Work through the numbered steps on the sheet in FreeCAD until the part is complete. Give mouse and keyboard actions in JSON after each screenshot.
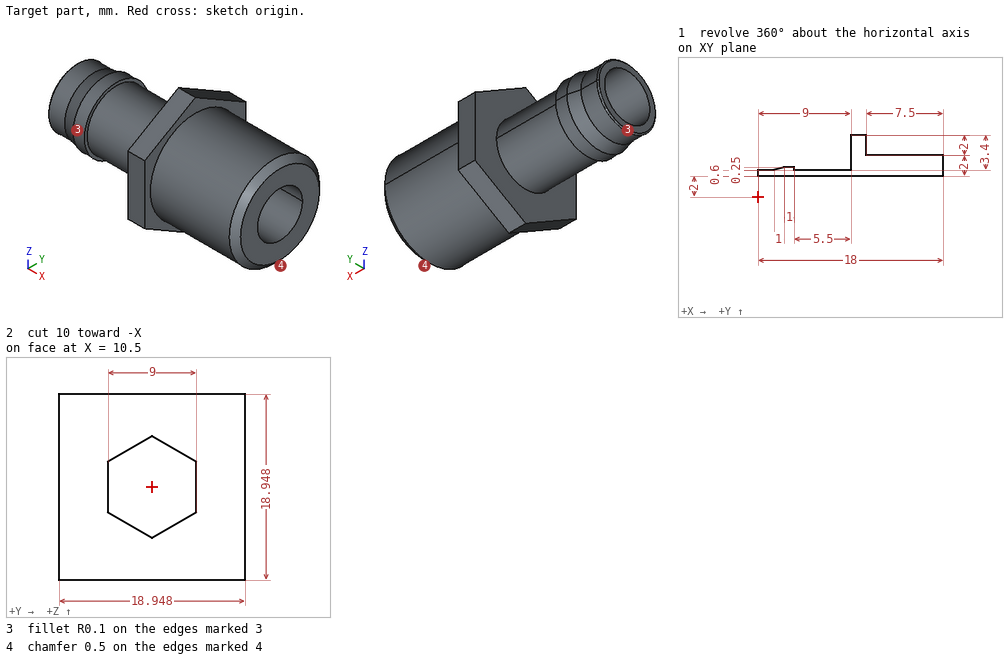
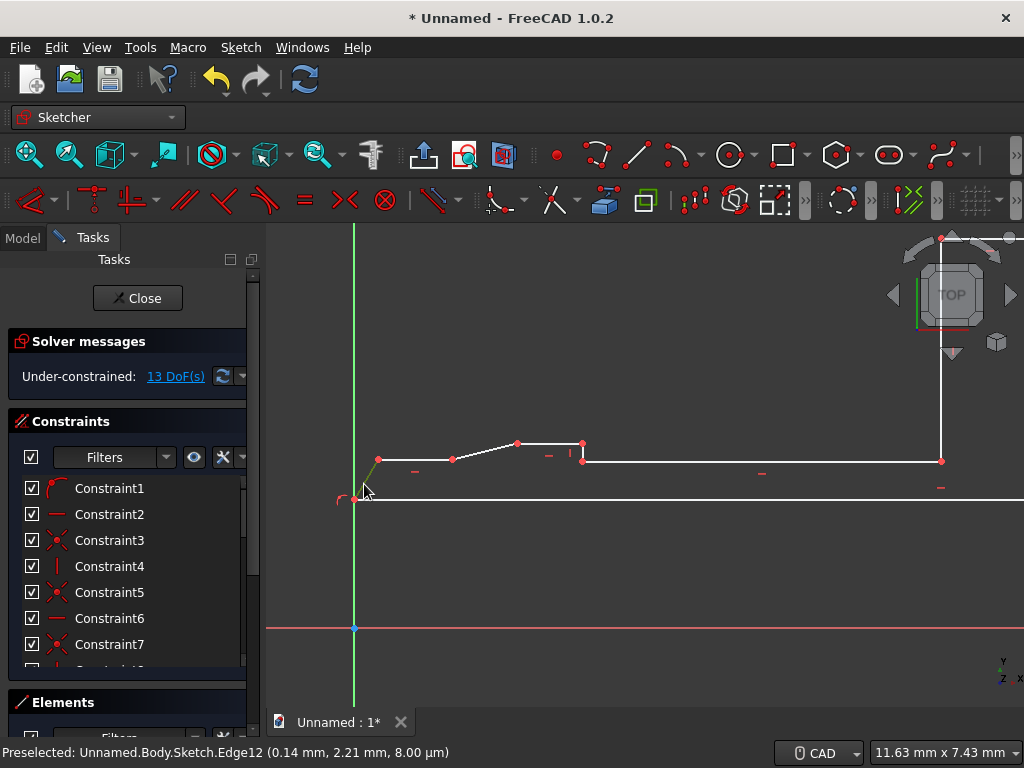
{"action": "key", "text": "v"}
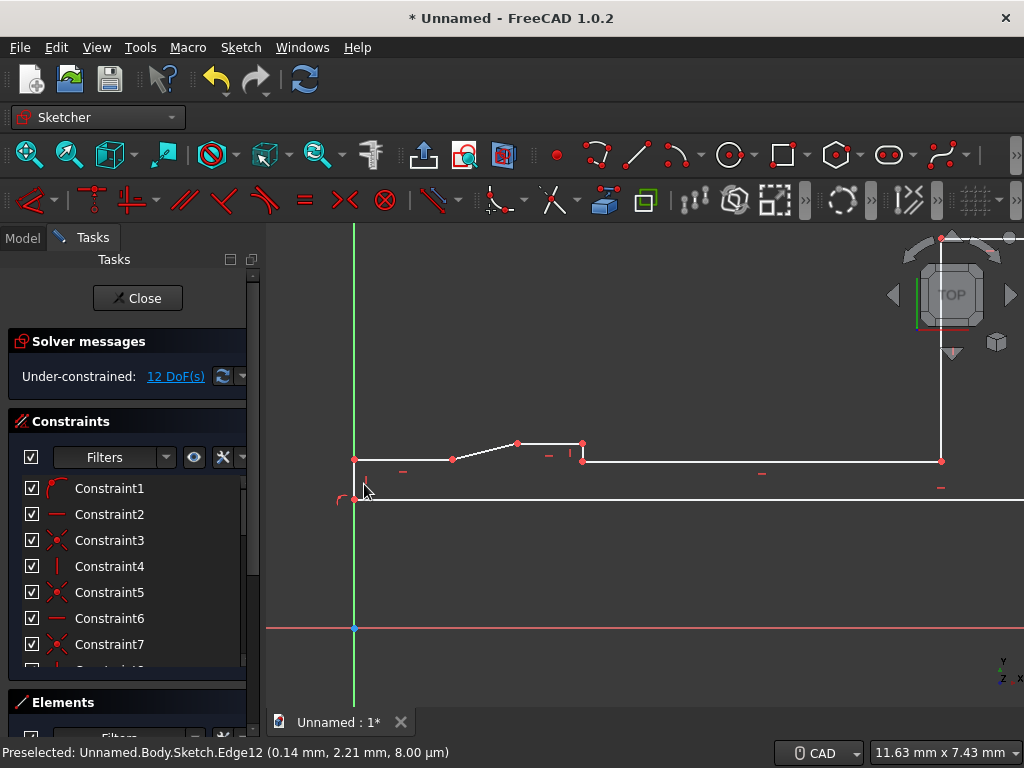
{"action": "scroll", "coordinate": [364, 484], "scroll_direction": "down", "scroll_amount": 5}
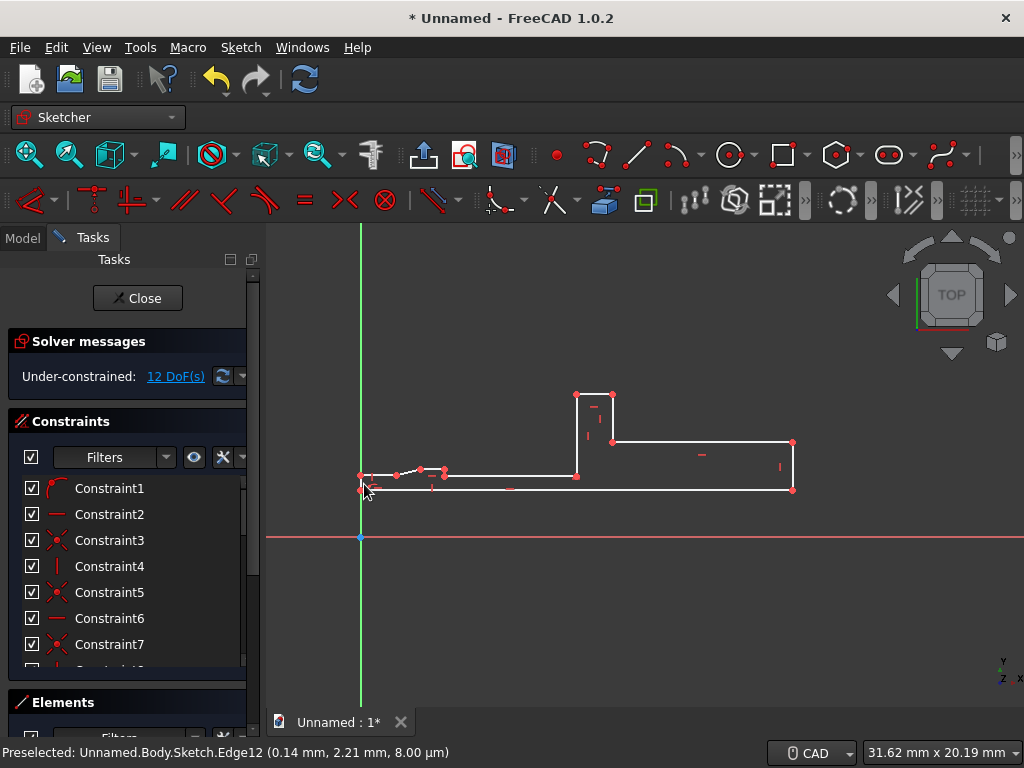
{"action": "left_click", "coordinate": [793, 476]}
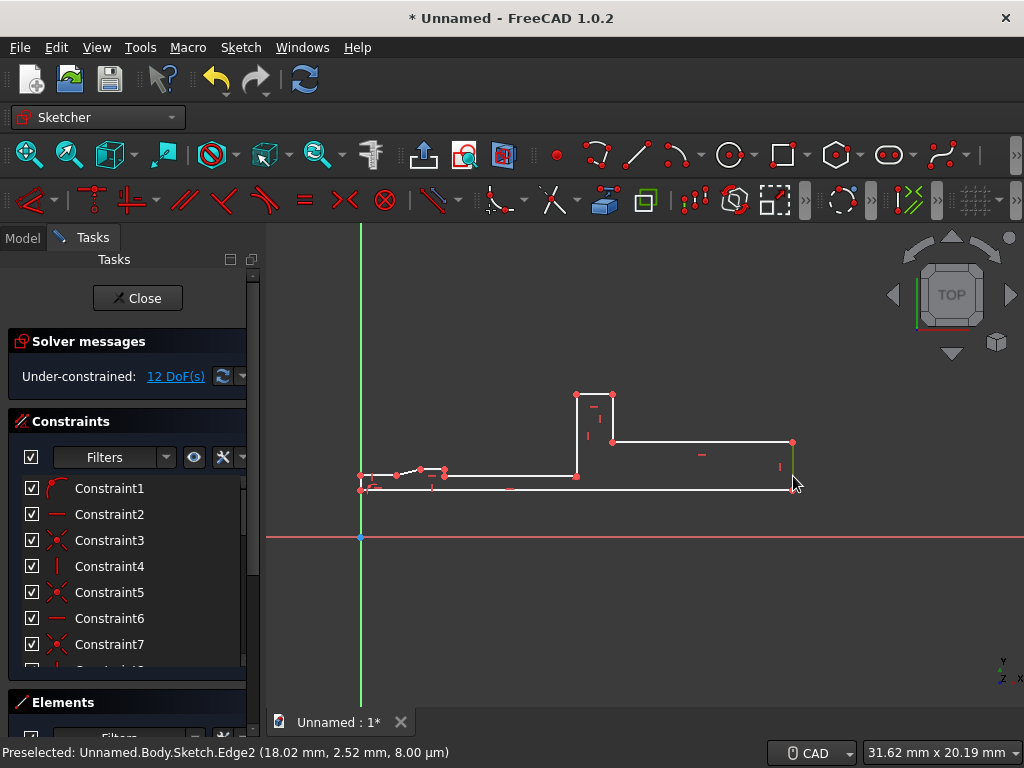
{"action": "key", "text": "i"}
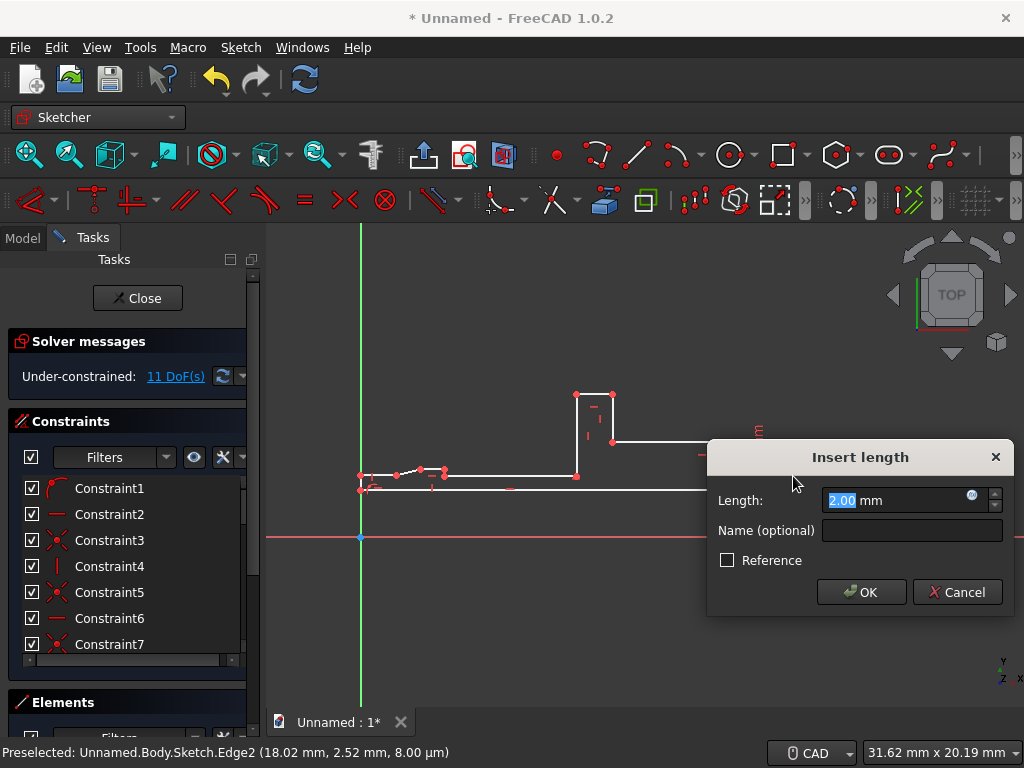
{"action": "type", "text": "2"}
{"action": "key", "text": "Return"}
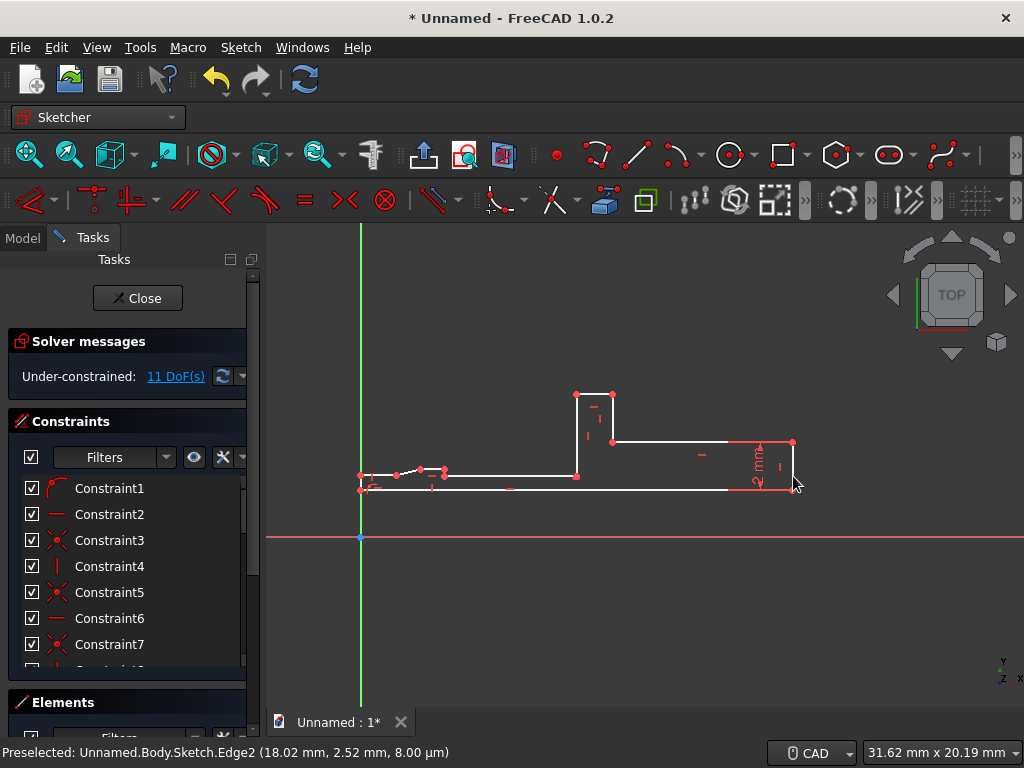
{"action": "left_click", "coordinate": [613, 428]}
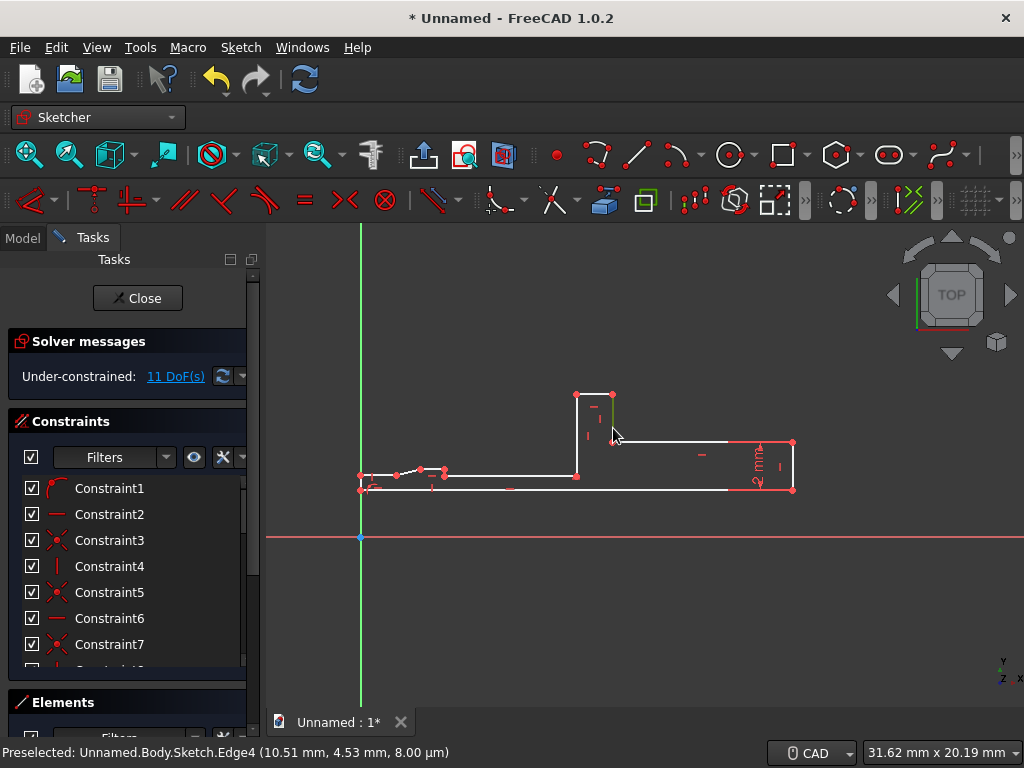
{"action": "key", "text": "i"}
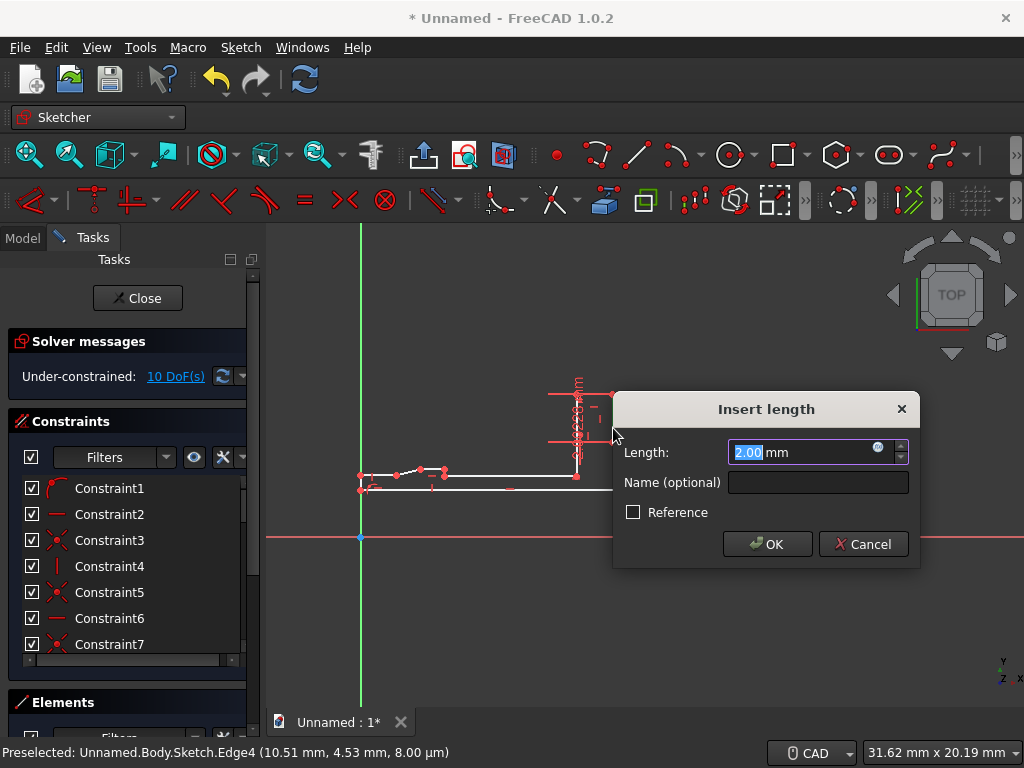
{"action": "type", "text": "2"}
{"action": "key", "text": "Return"}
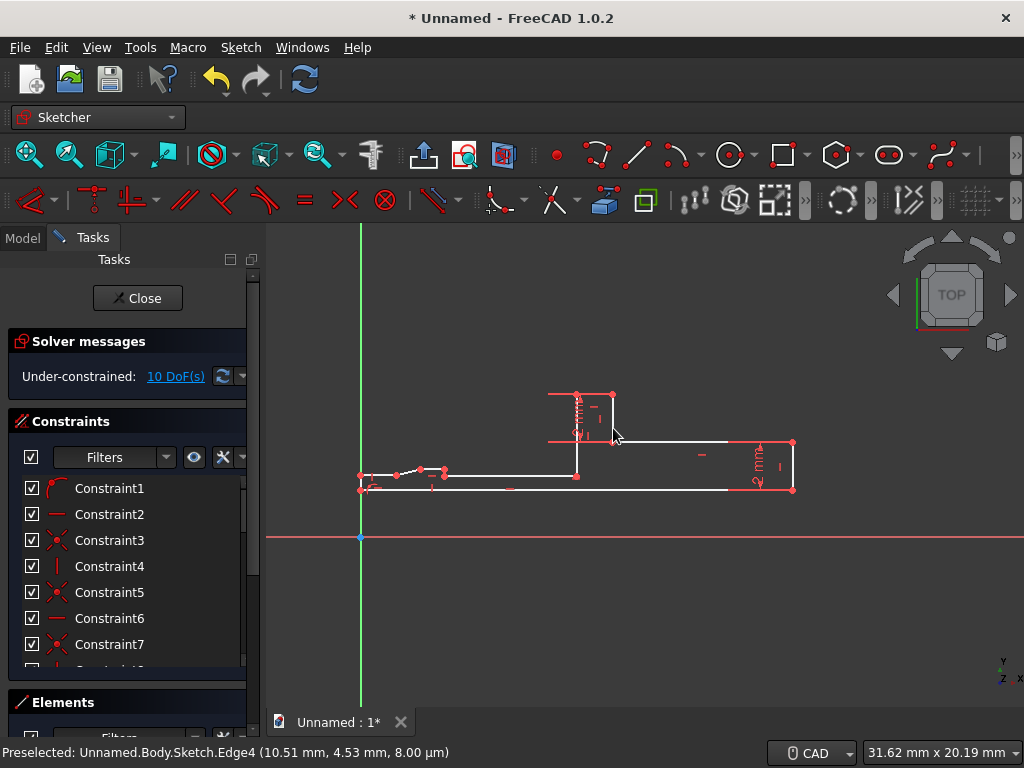
{"action": "scroll", "coordinate": [435, 469], "scroll_direction": "up", "scroll_amount": 3}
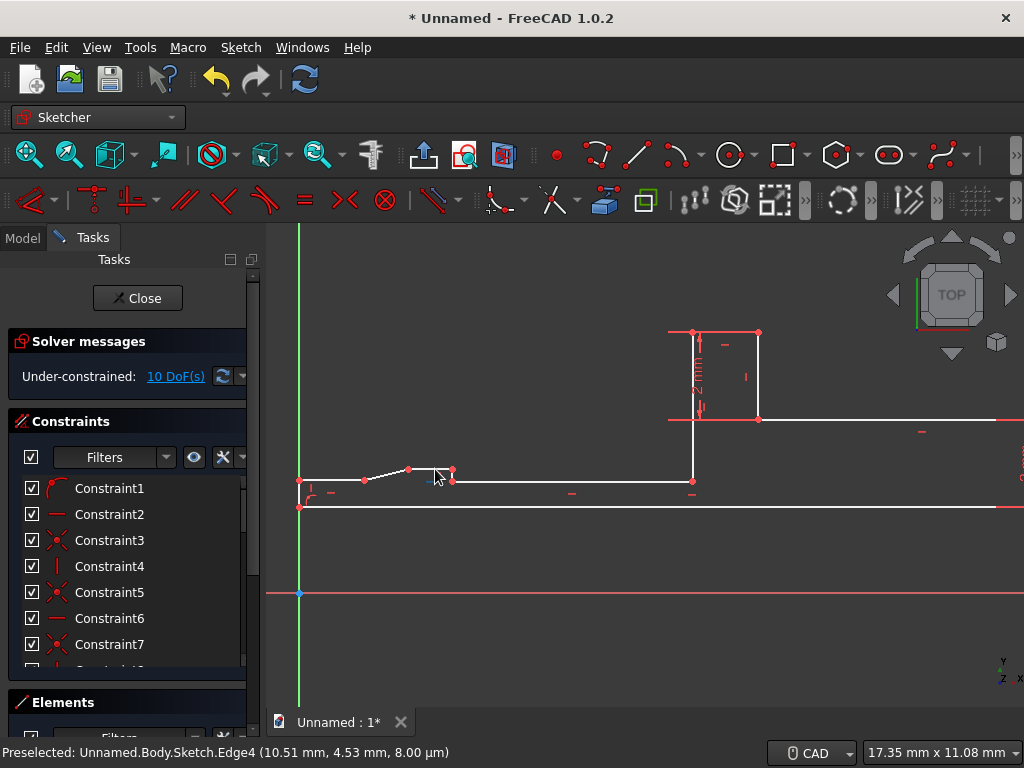
{"action": "left_click", "coordinate": [426, 469]}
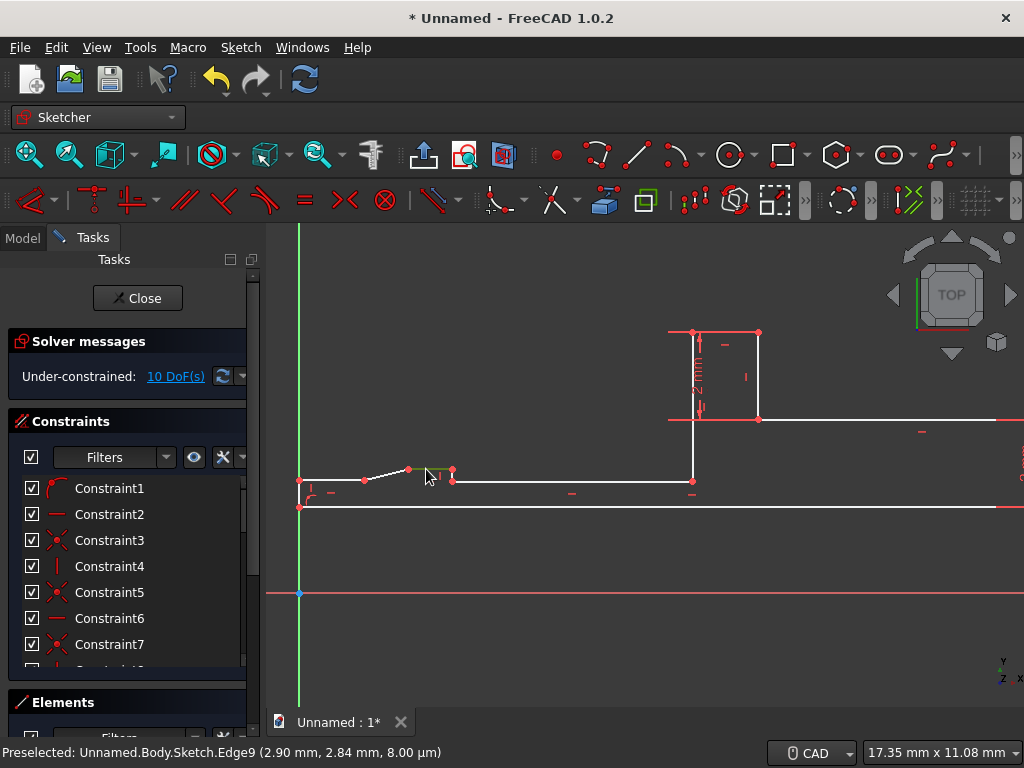
{"action": "left_click", "coordinate": [56, 200]}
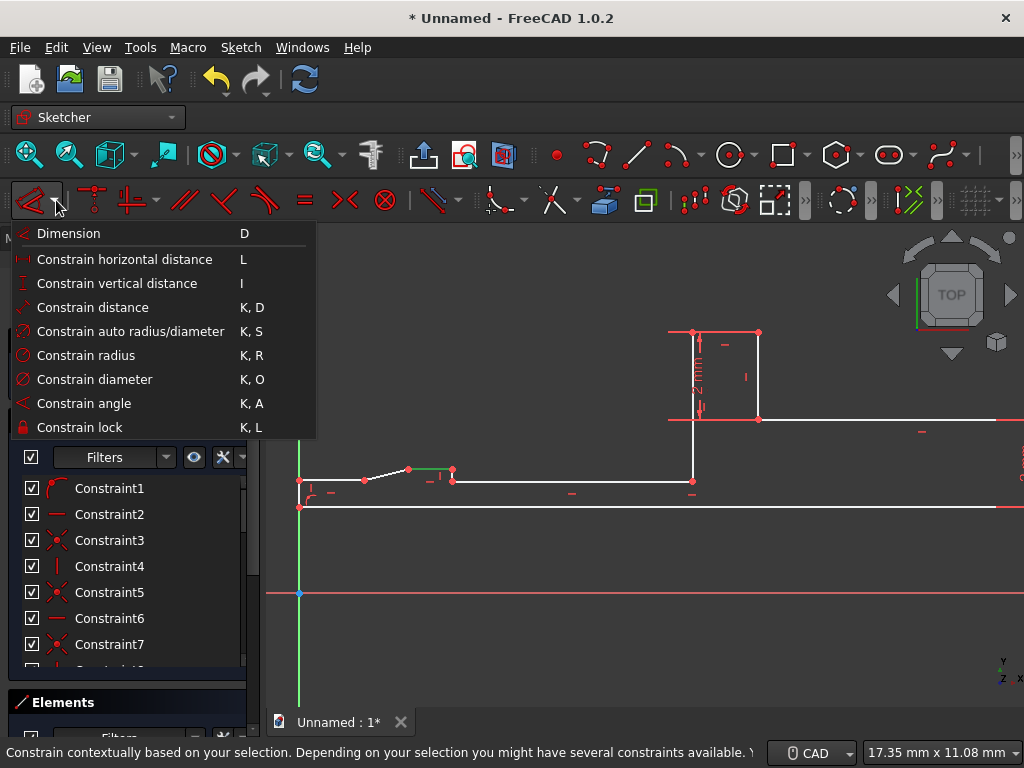
{"action": "left_click", "coordinate": [164, 259]}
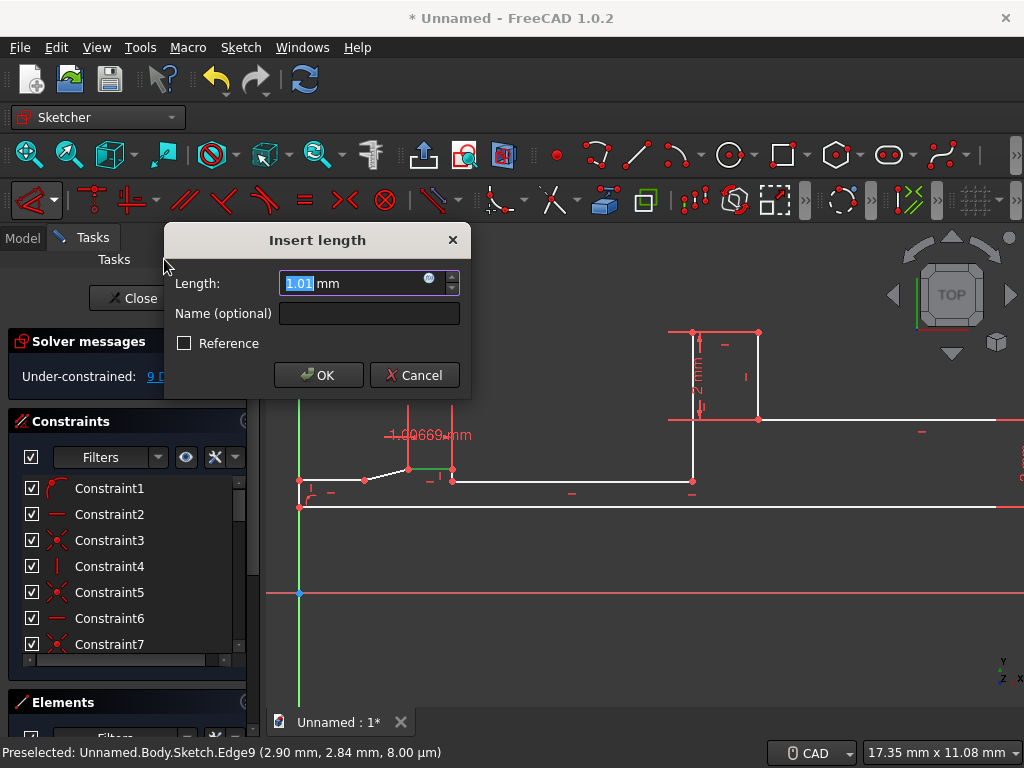
{"action": "type", "text": "1"}
{"action": "key", "text": "Return"}